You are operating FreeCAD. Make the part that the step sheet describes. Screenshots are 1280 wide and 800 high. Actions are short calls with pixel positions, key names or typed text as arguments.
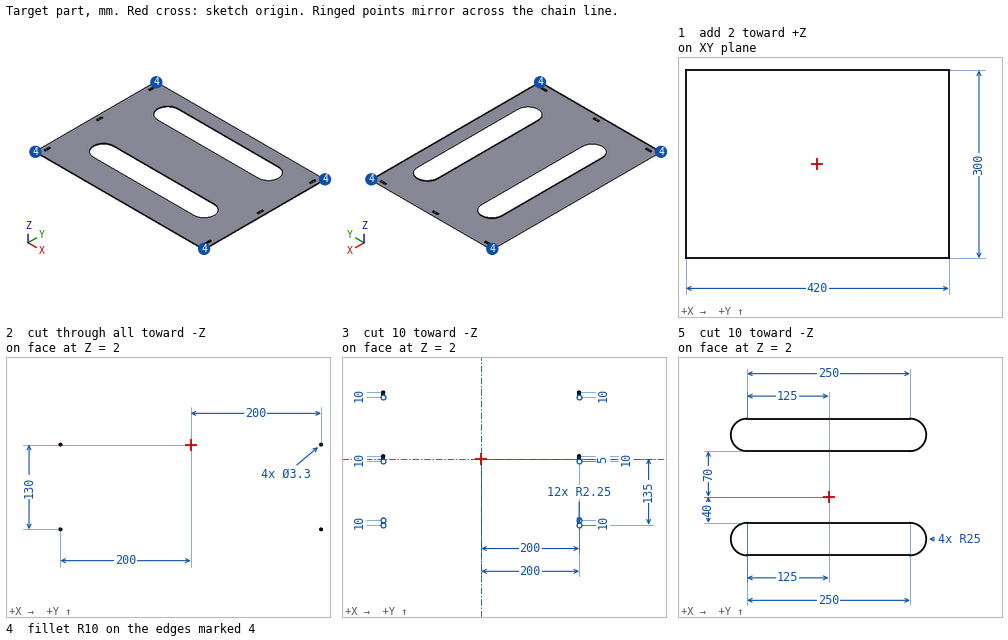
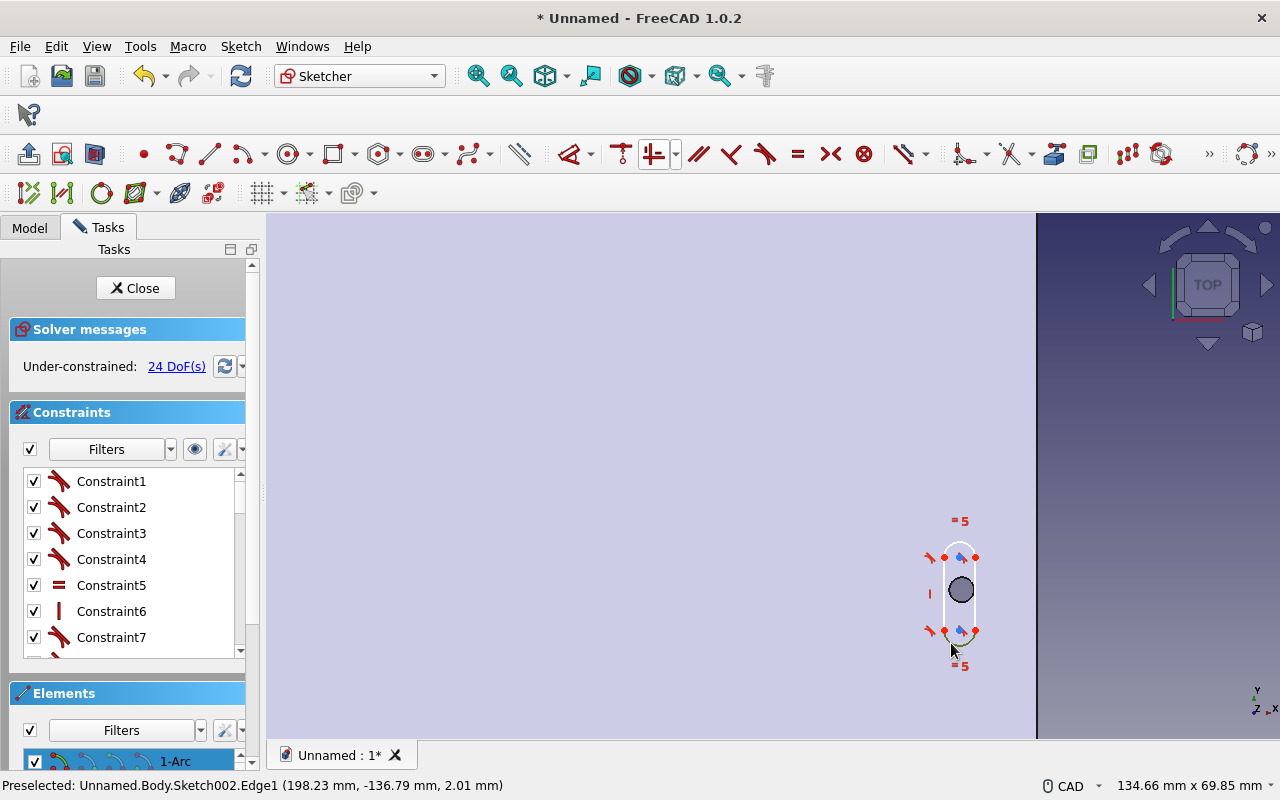
scroll(952, 647, down, 9)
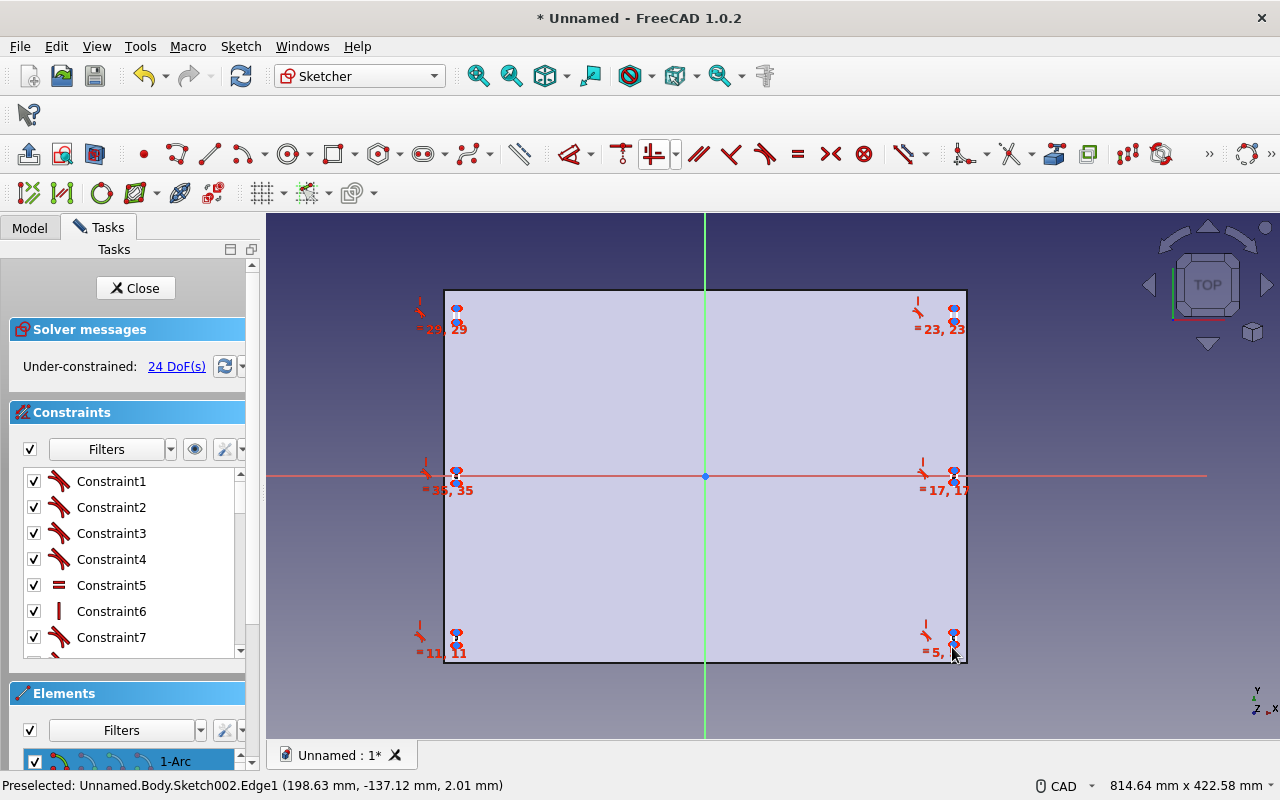
scroll(455, 648, up, 9)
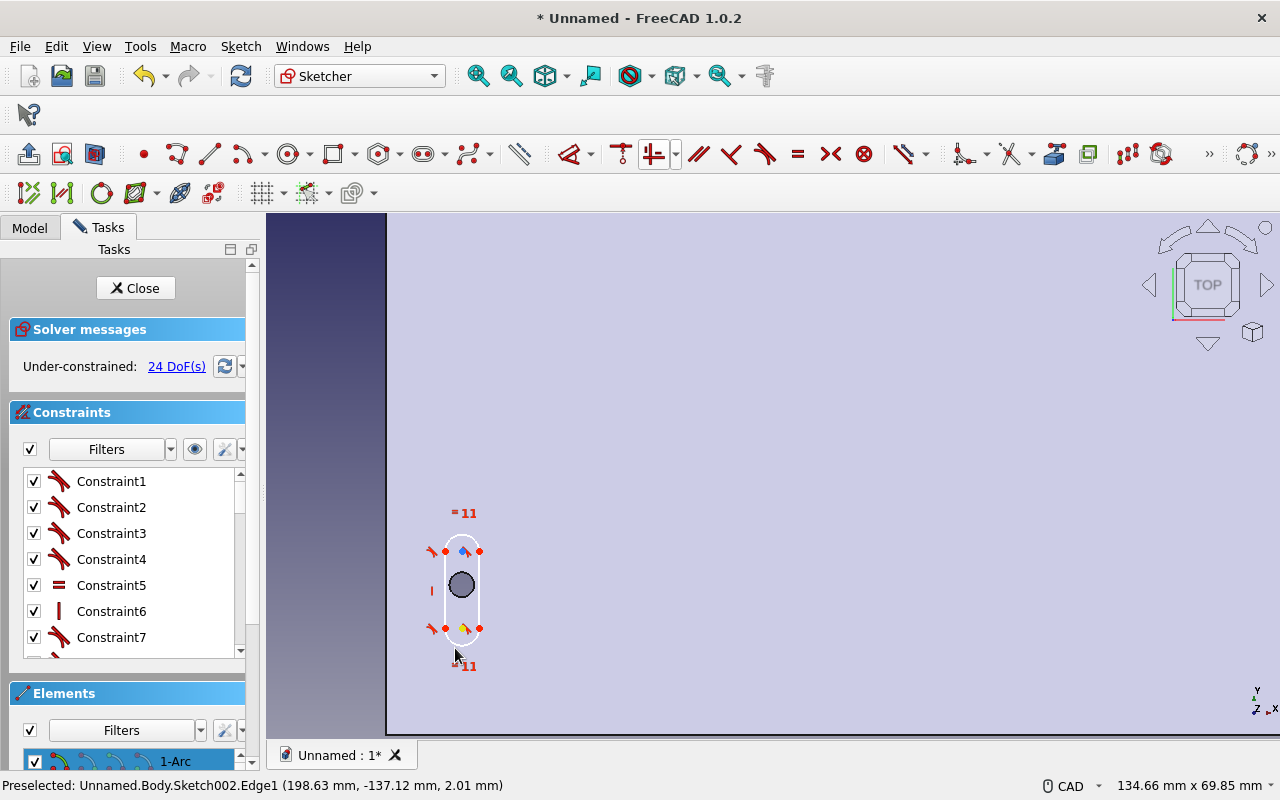
click(452, 642)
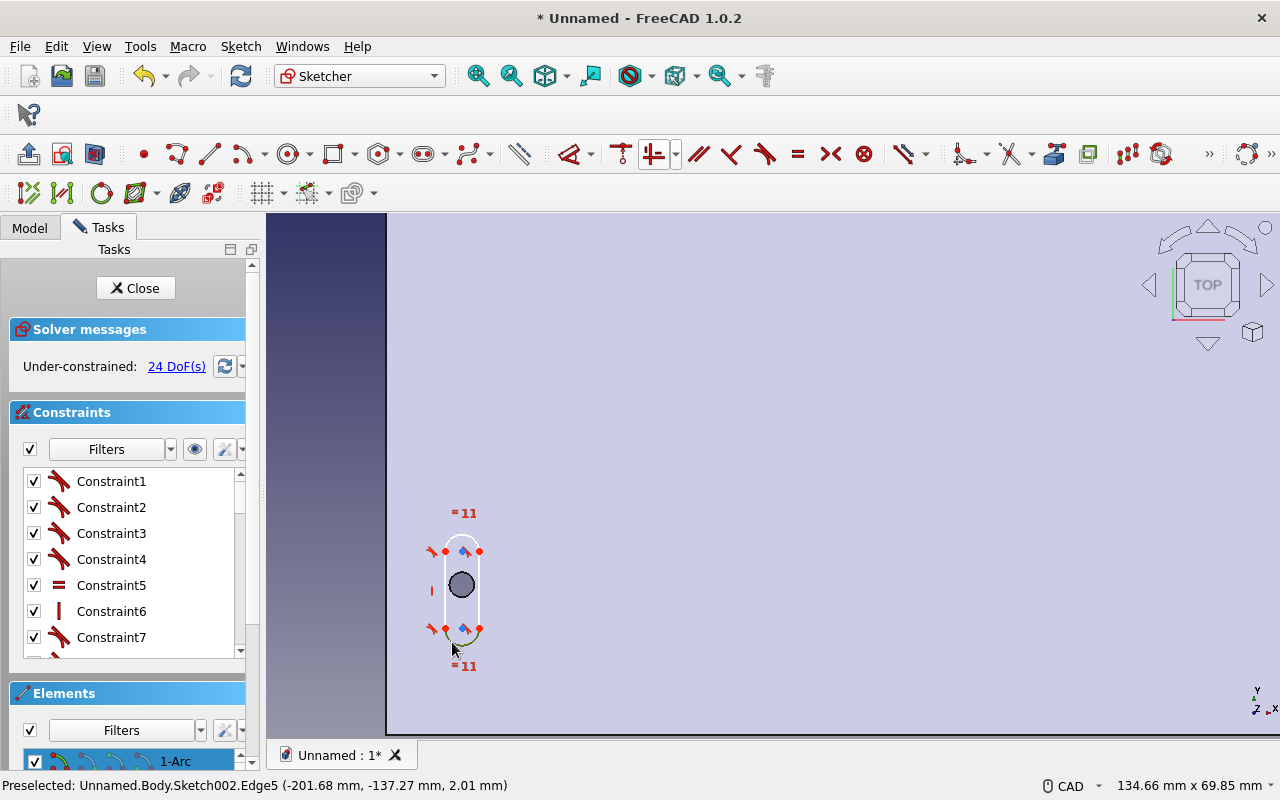
scroll(454, 648, down, 9)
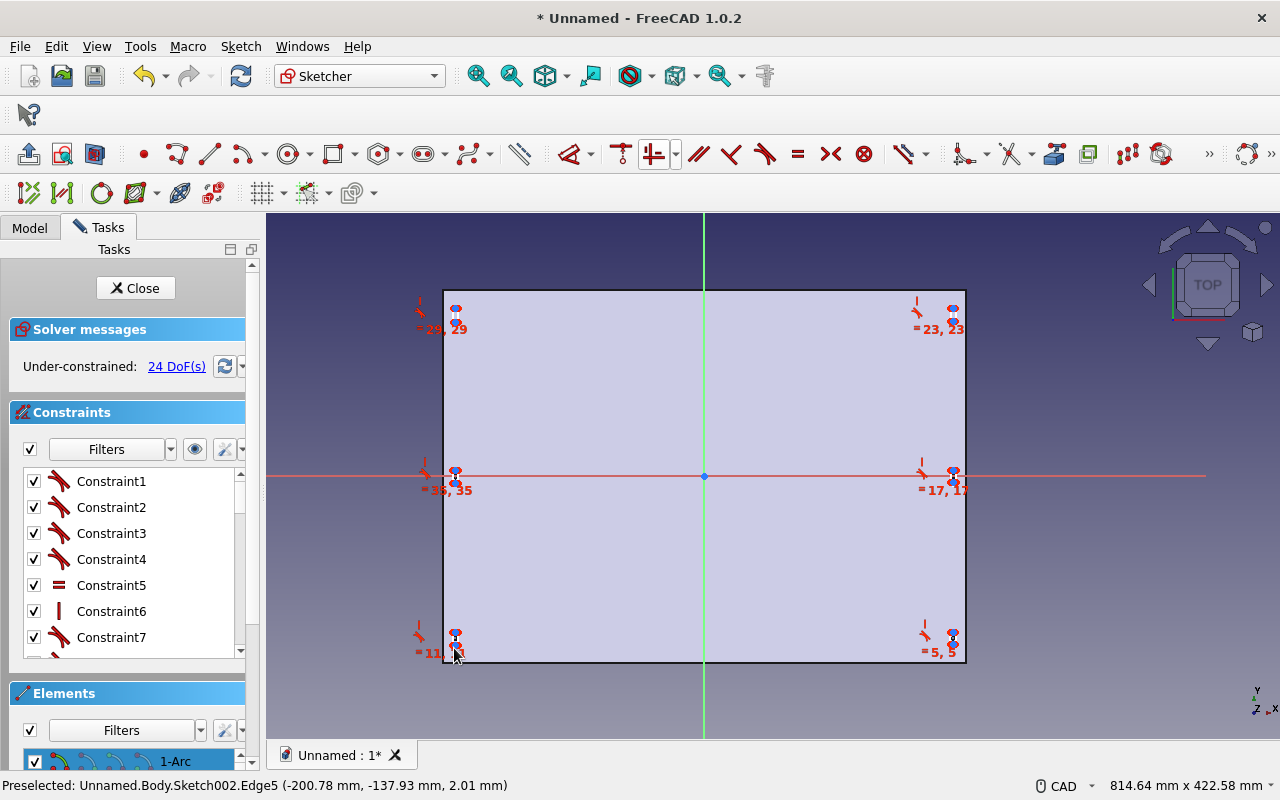
scroll(952, 485, up, 9)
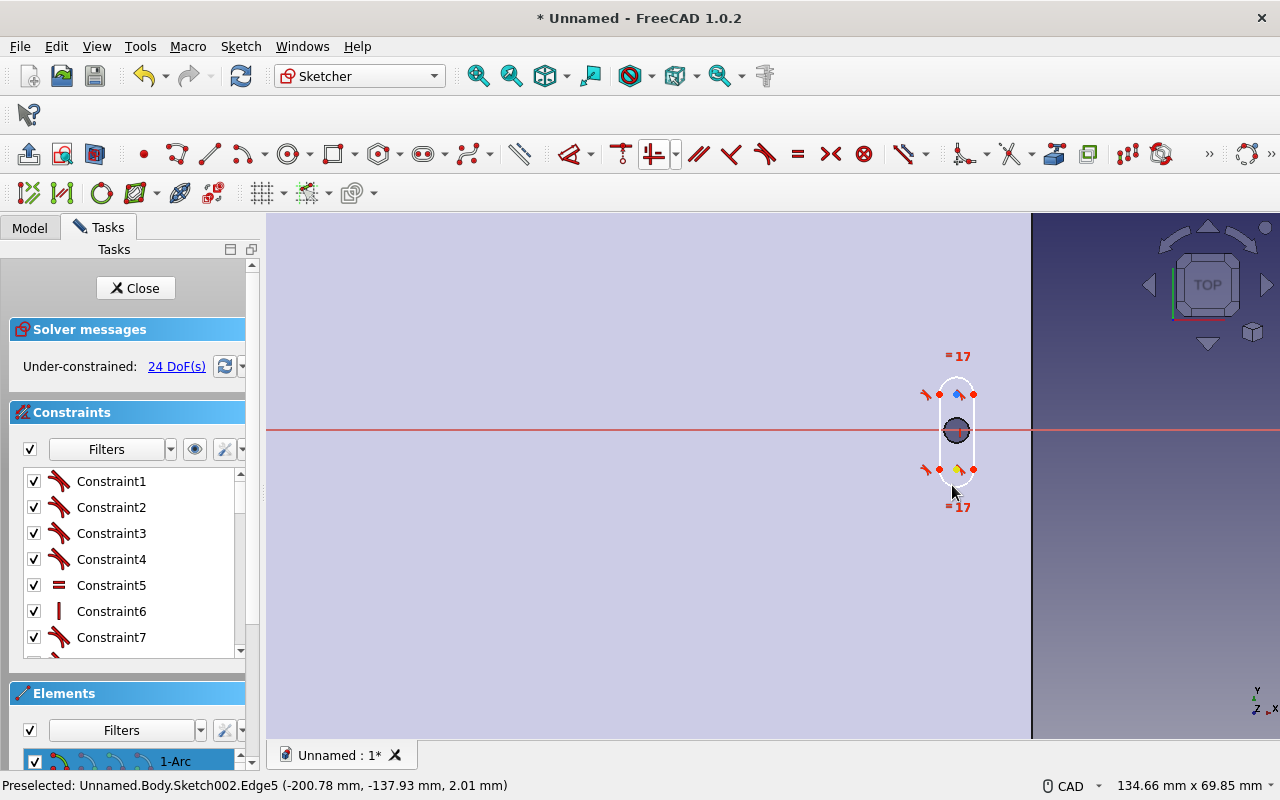
click(947, 484)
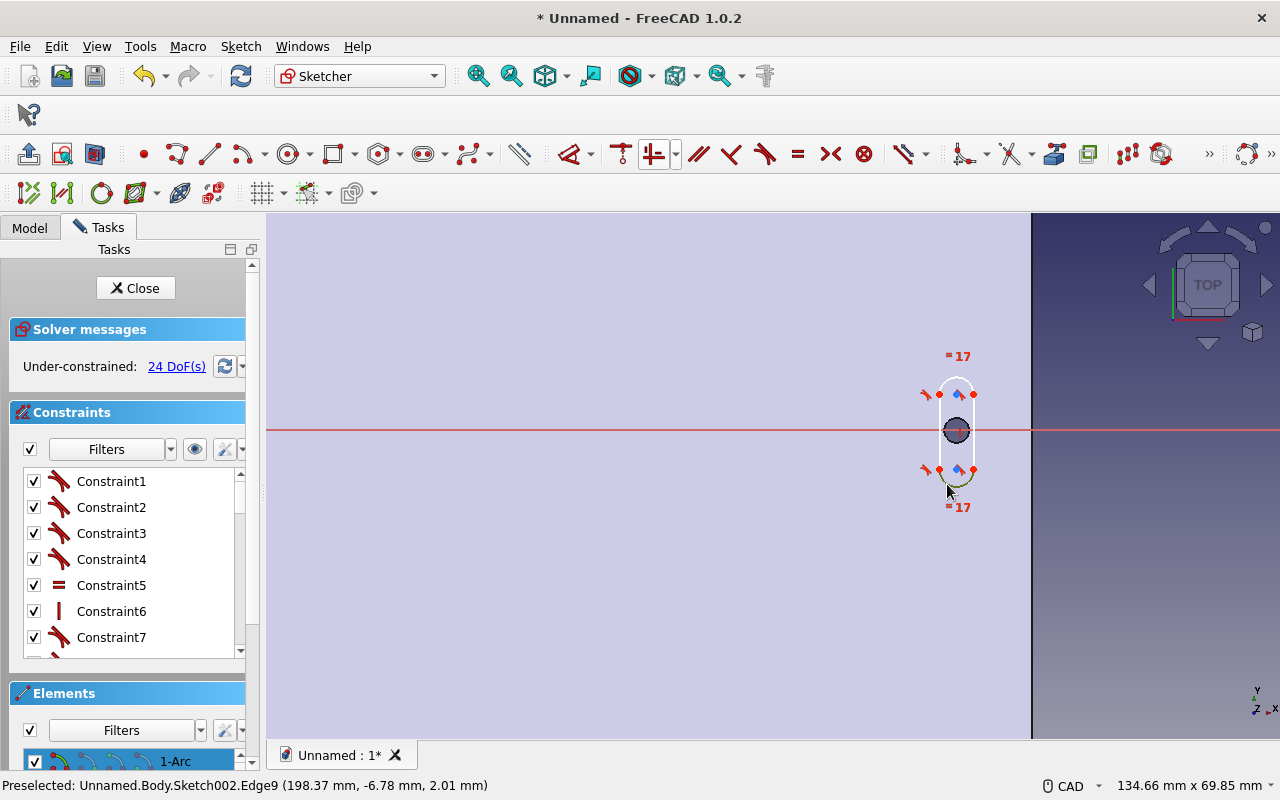
scroll(953, 485, down, 9)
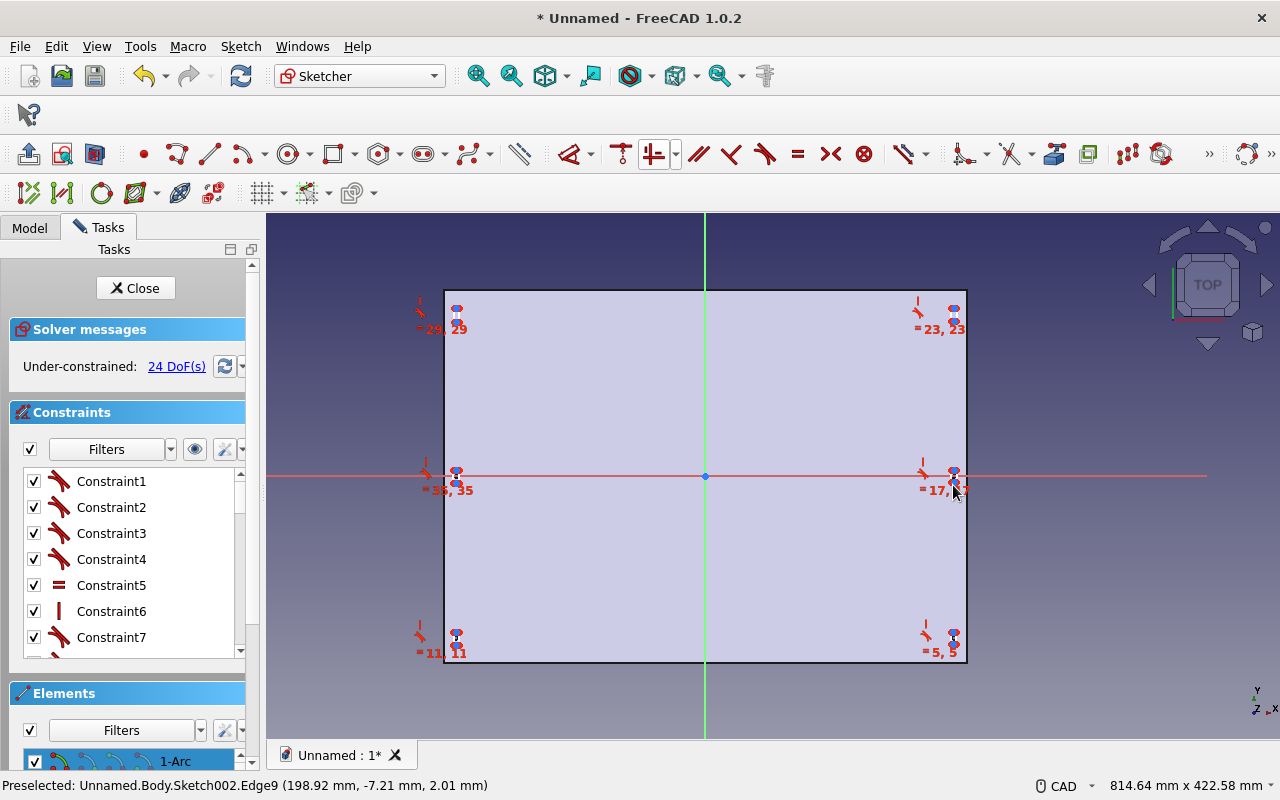
scroll(953, 324, up, 9)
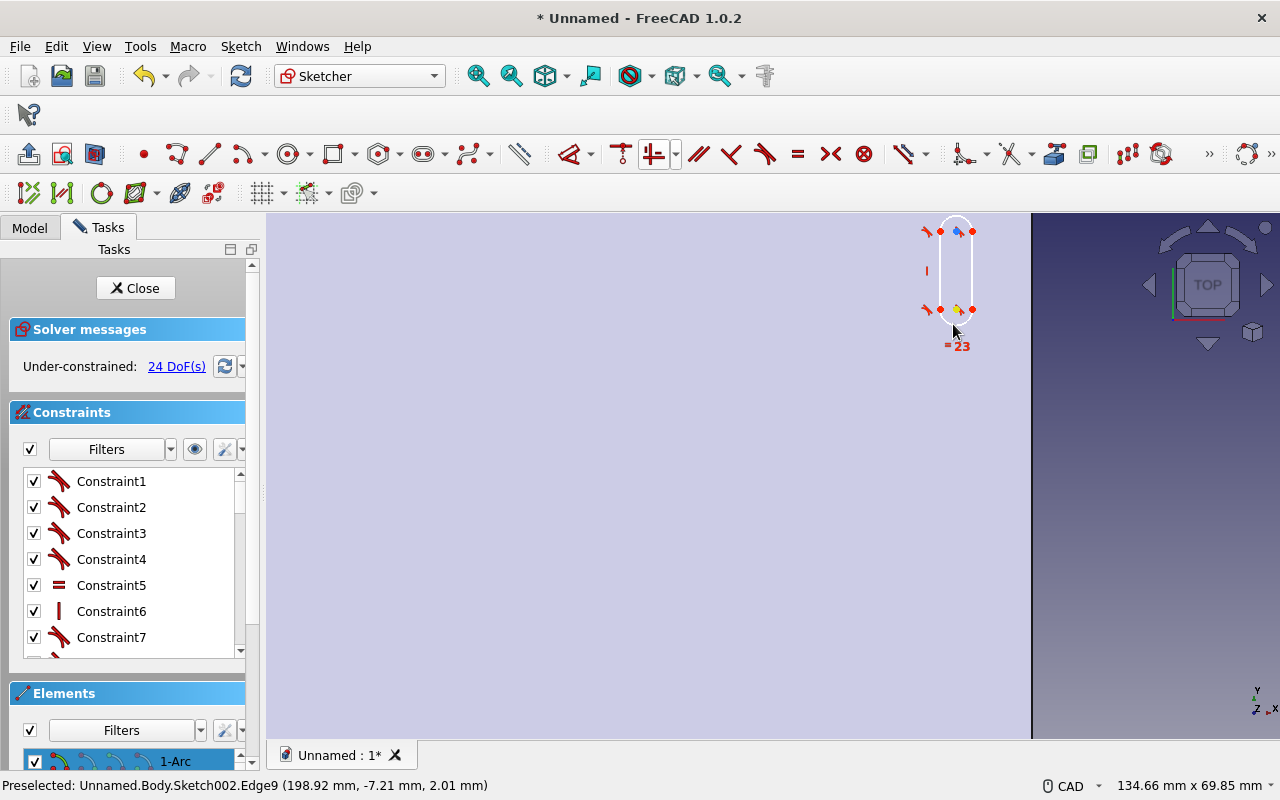
click(947, 322)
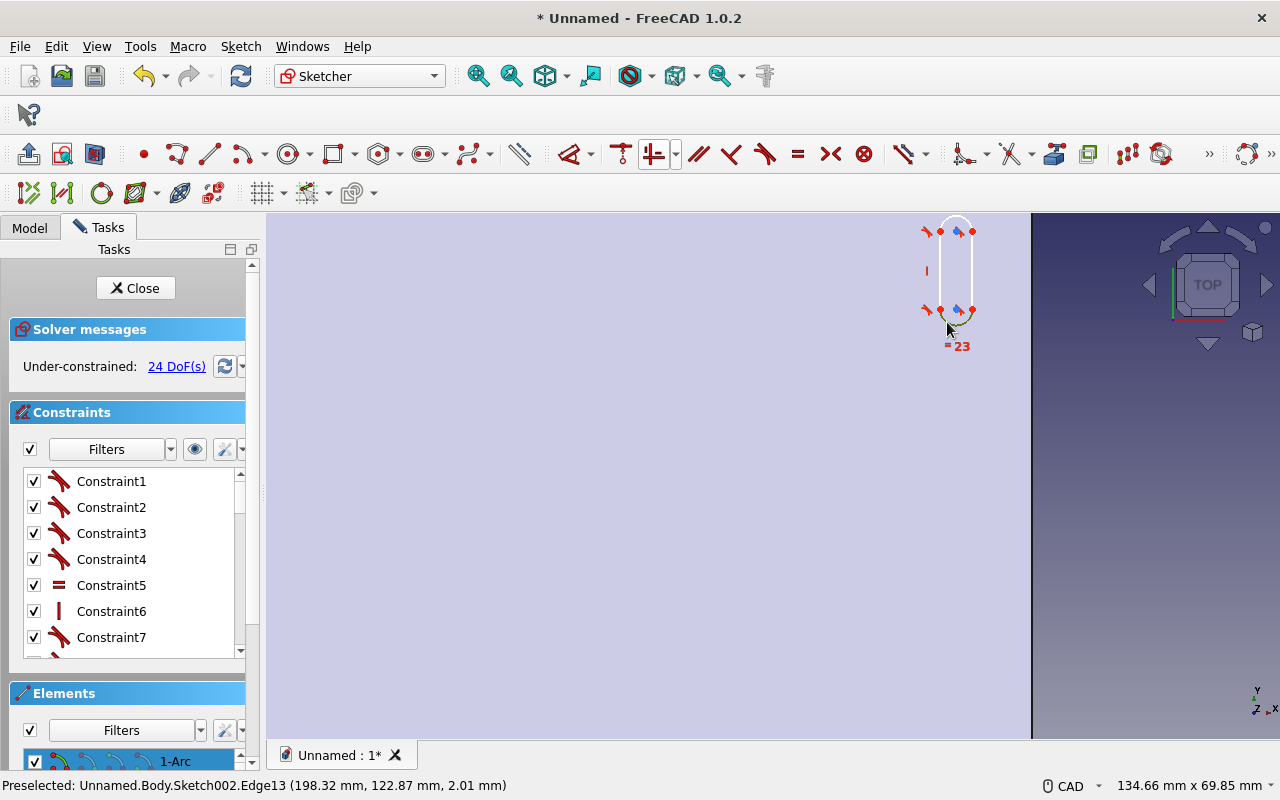
scroll(953, 324, down, 9)